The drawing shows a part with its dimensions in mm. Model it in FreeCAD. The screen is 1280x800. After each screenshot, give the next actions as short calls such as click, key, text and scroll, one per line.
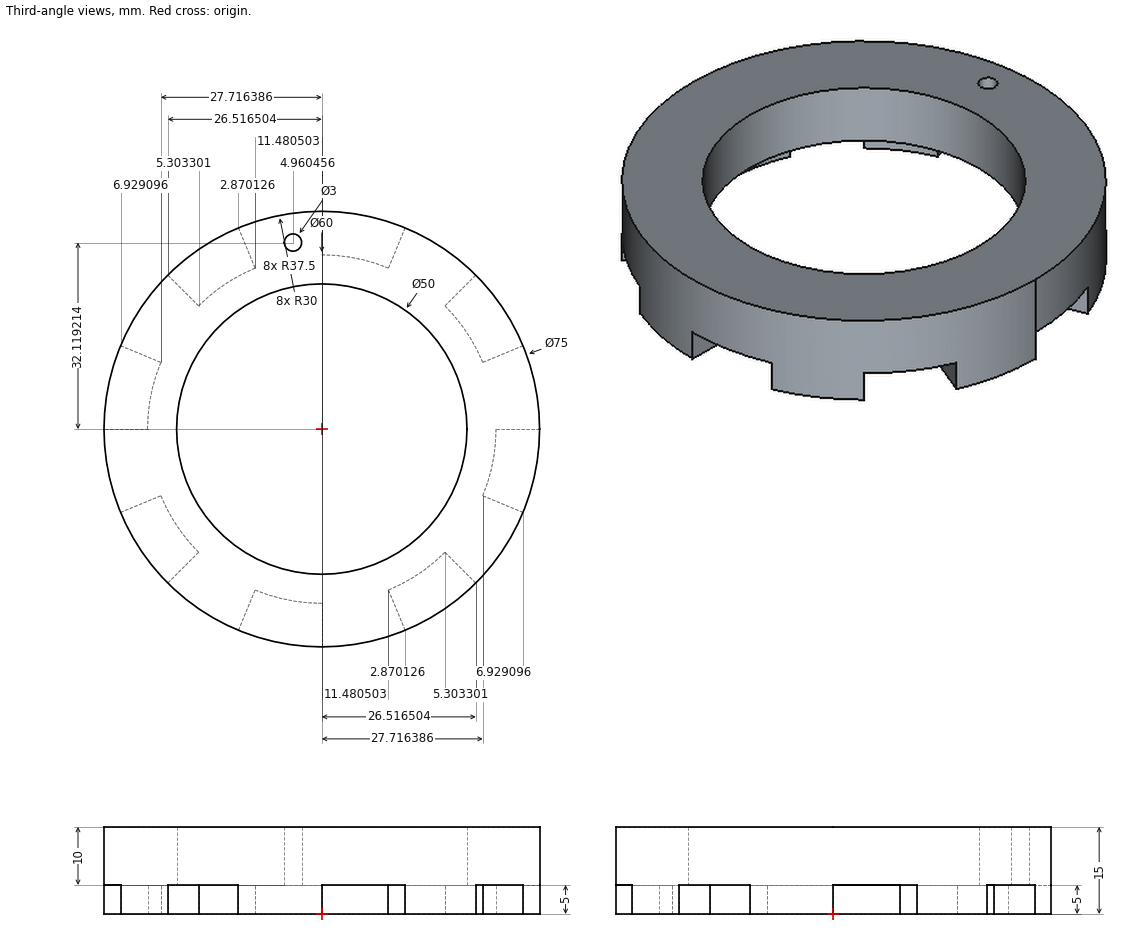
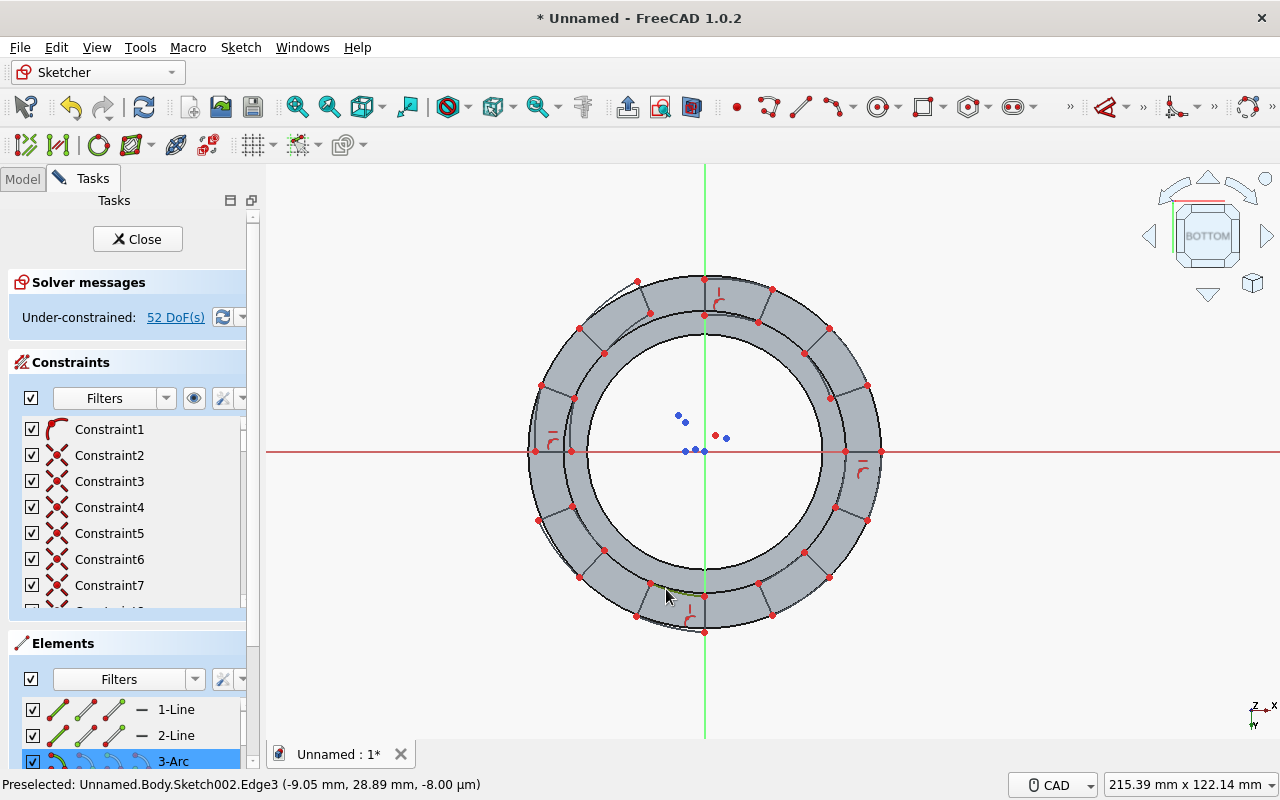
click(859, 367)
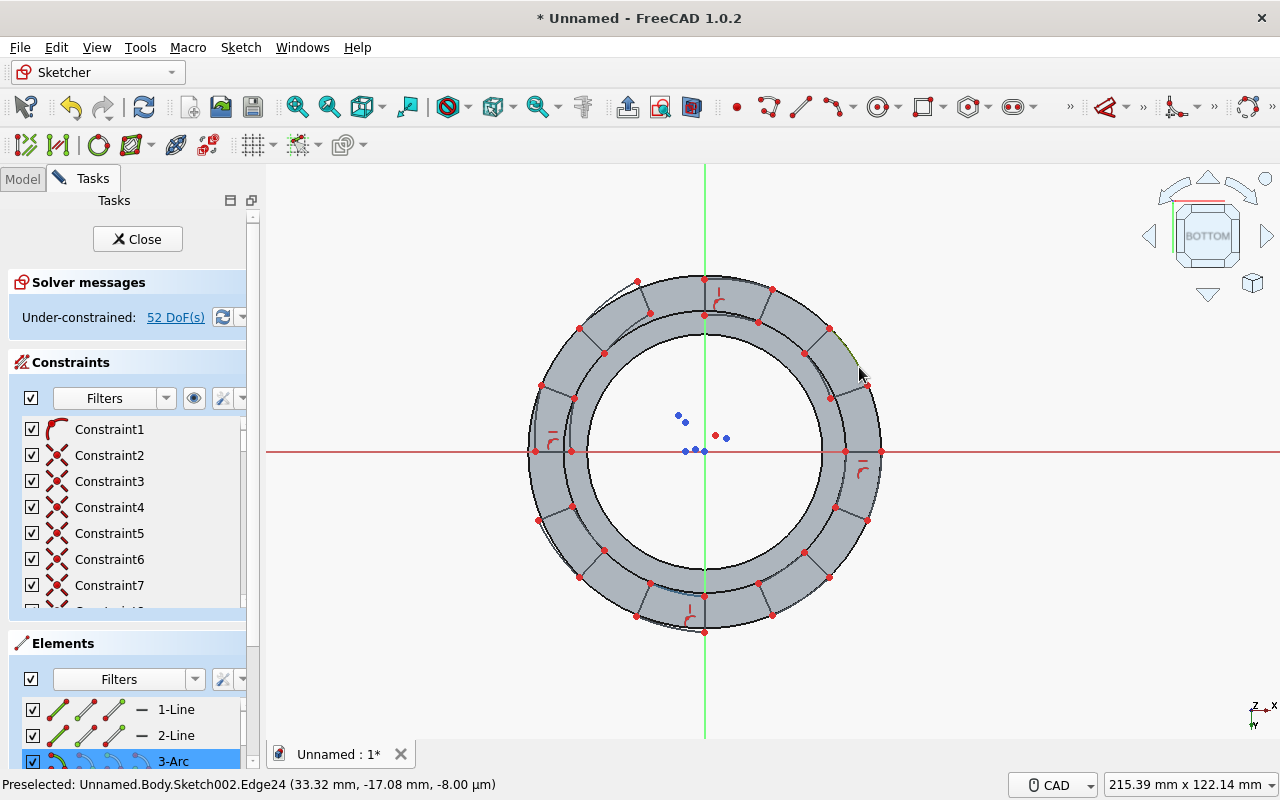
key(c)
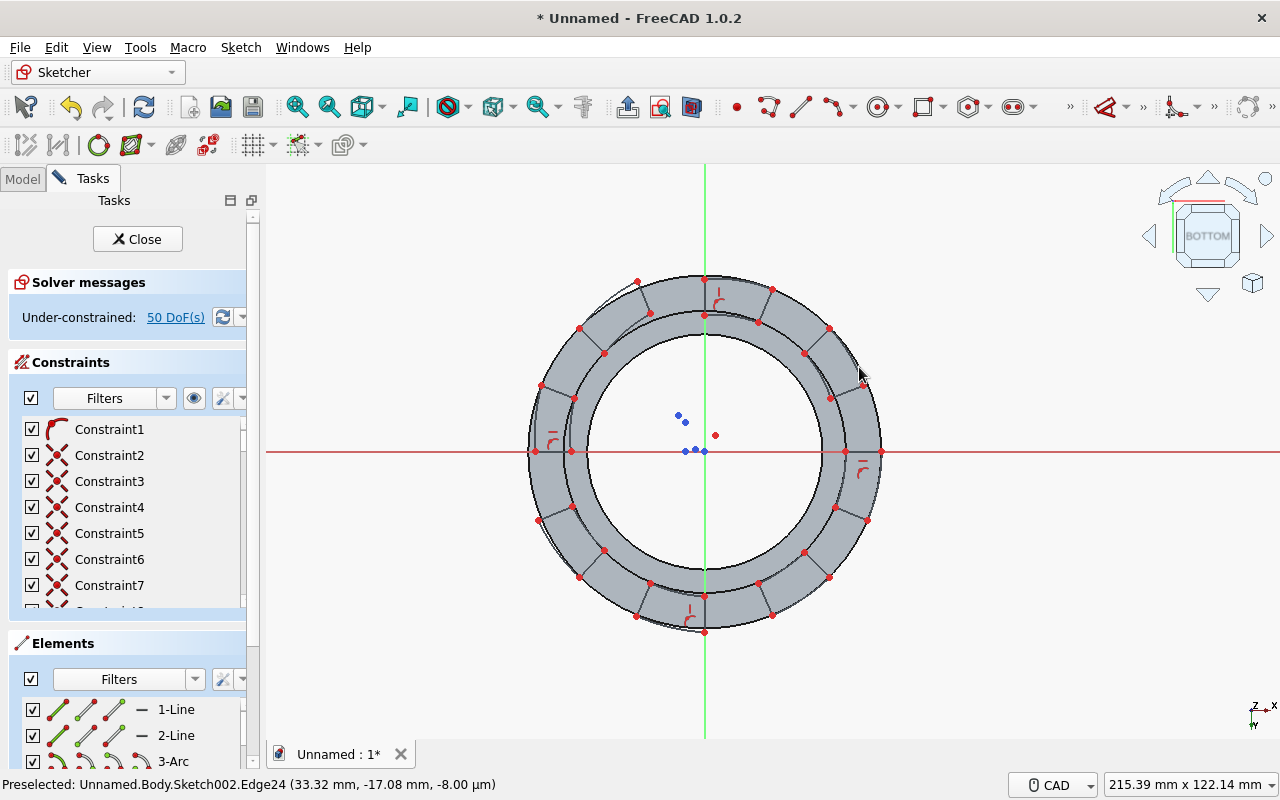
click(666, 589)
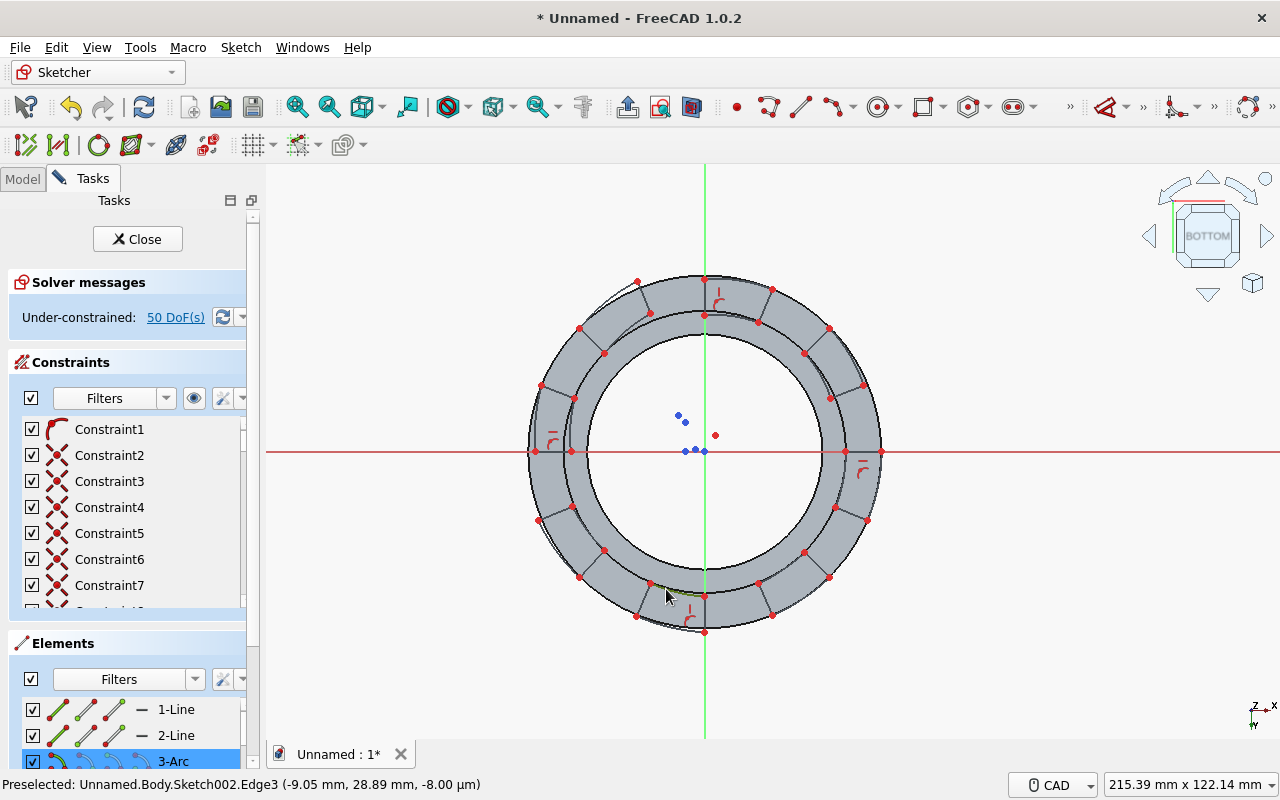
click(841, 491)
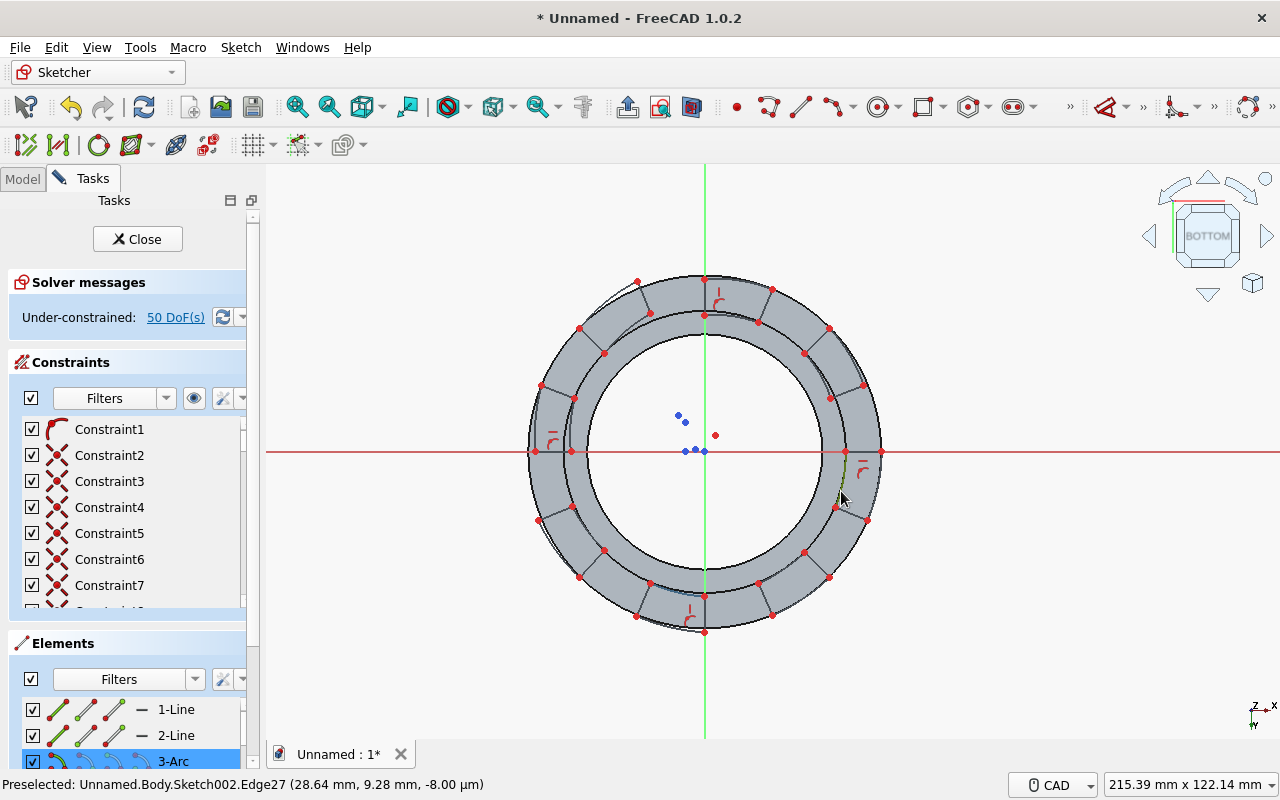
key(c)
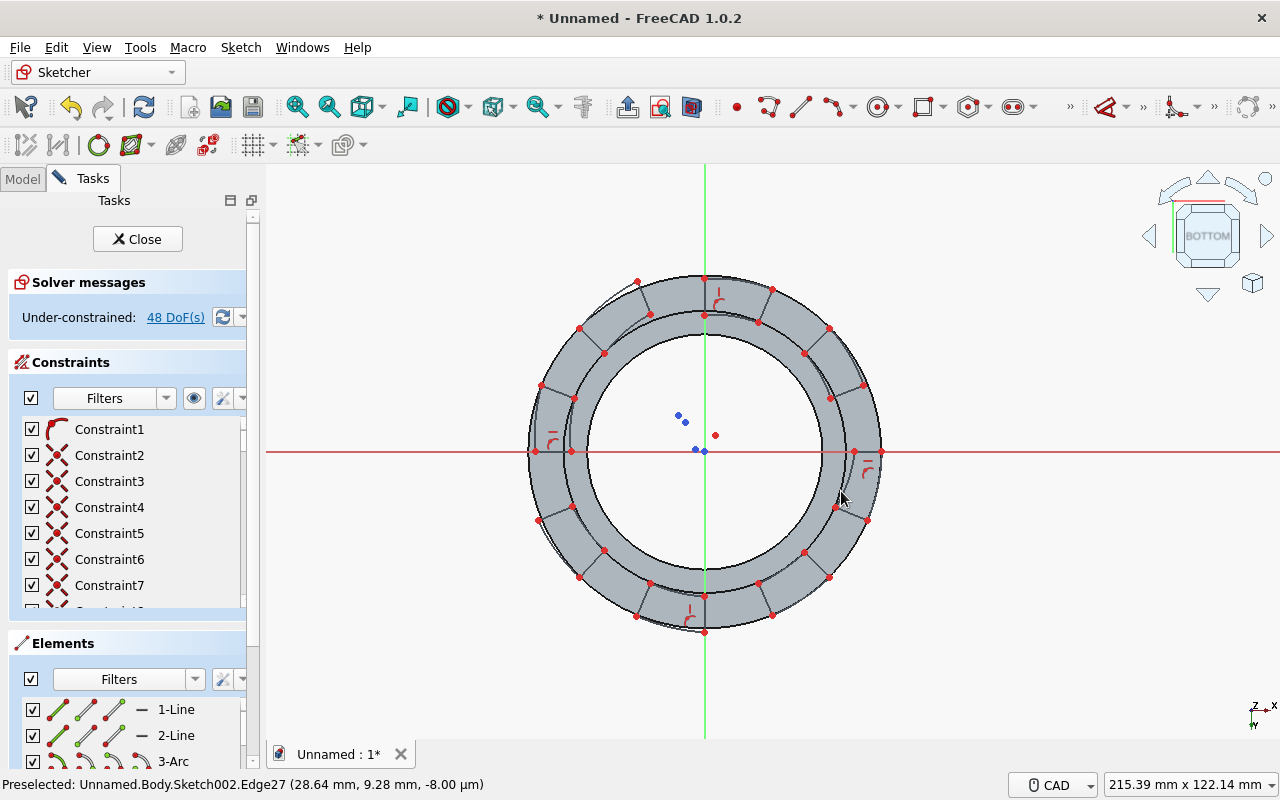
click(666, 589)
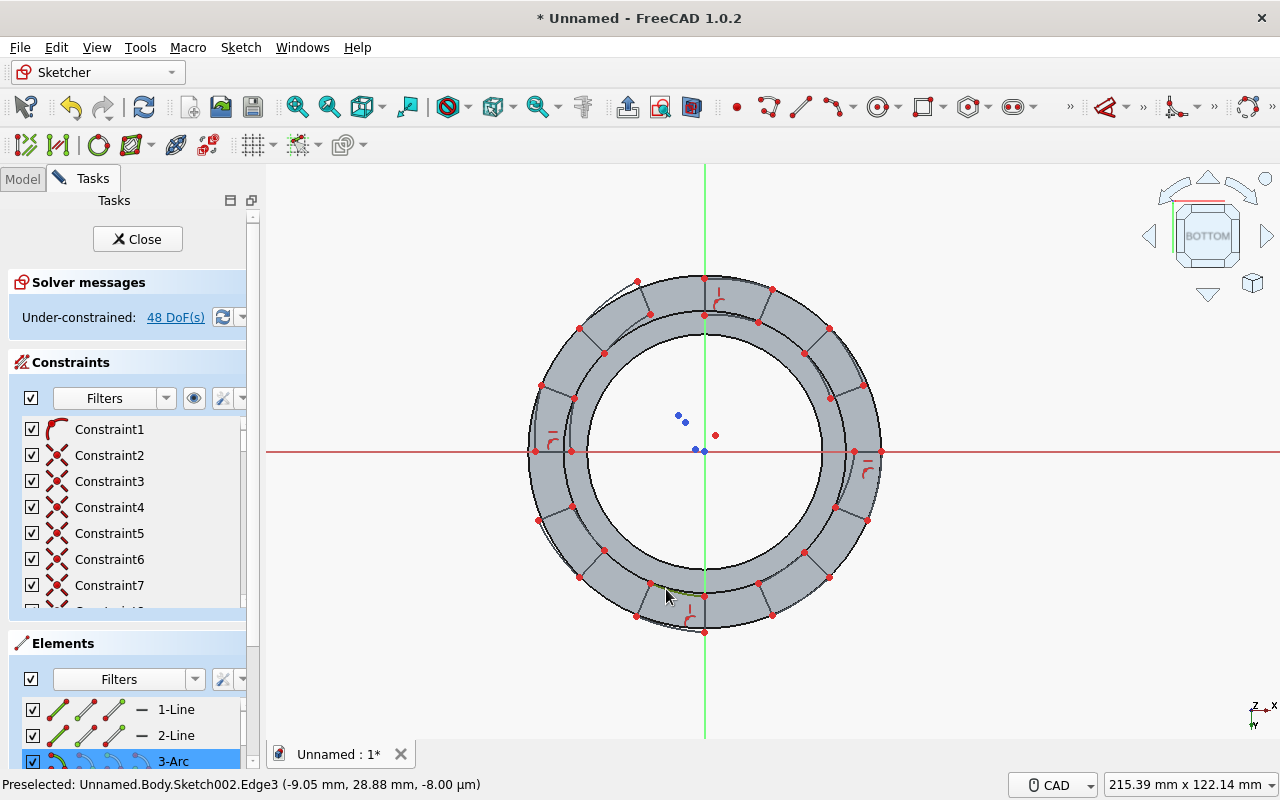
click(875, 501)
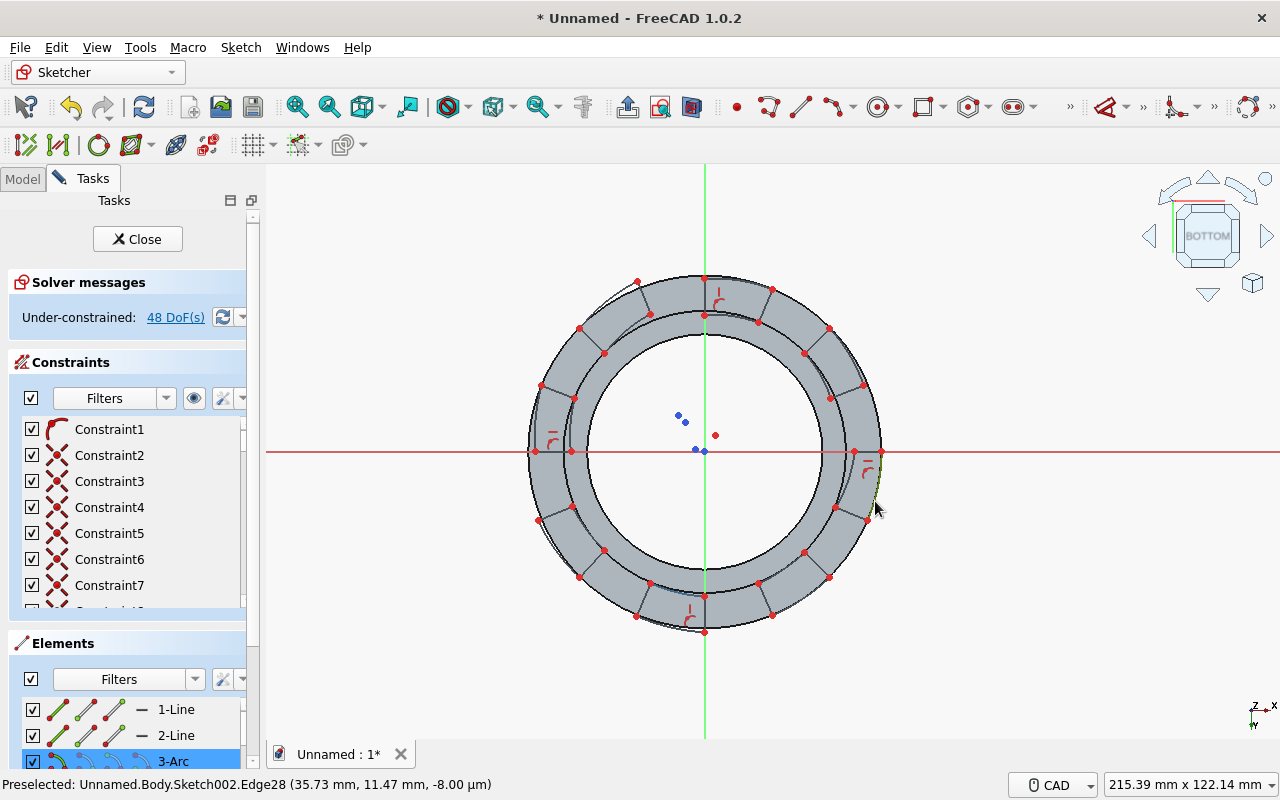
key(c)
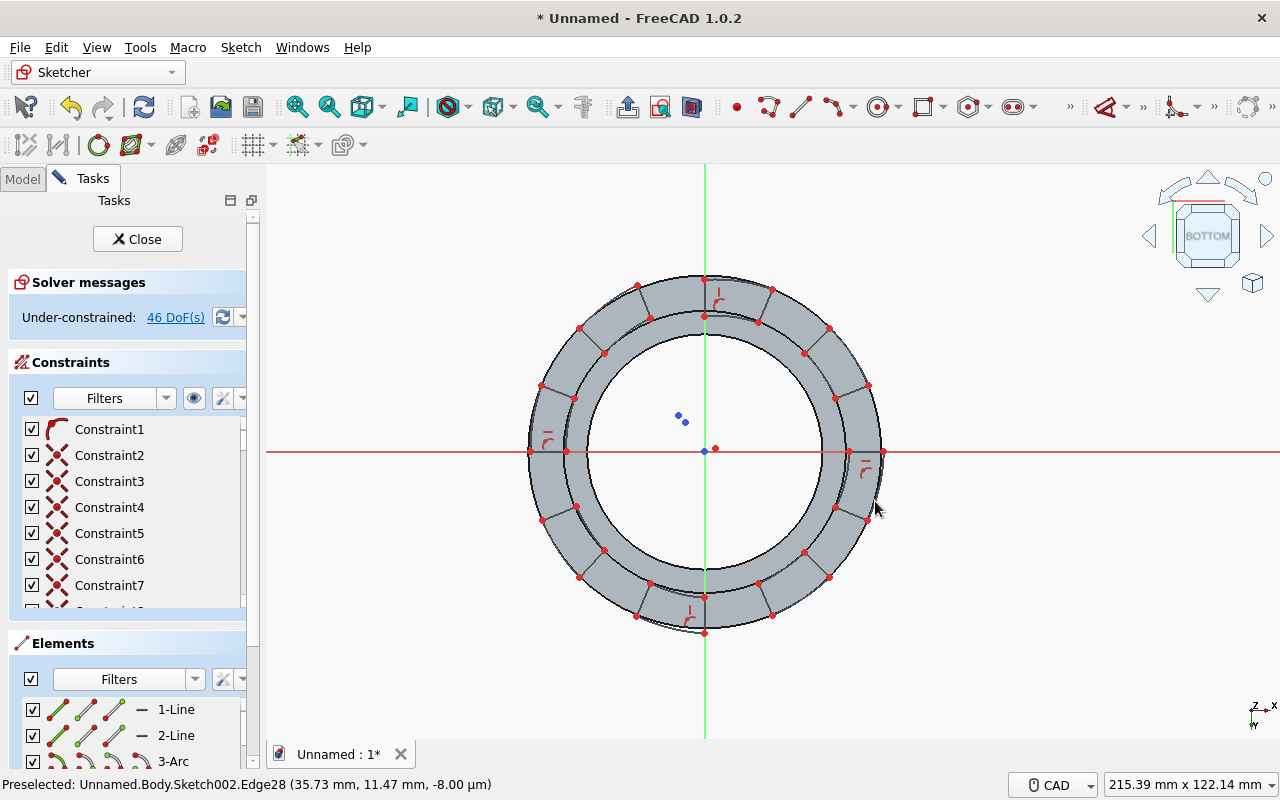
click(666, 590)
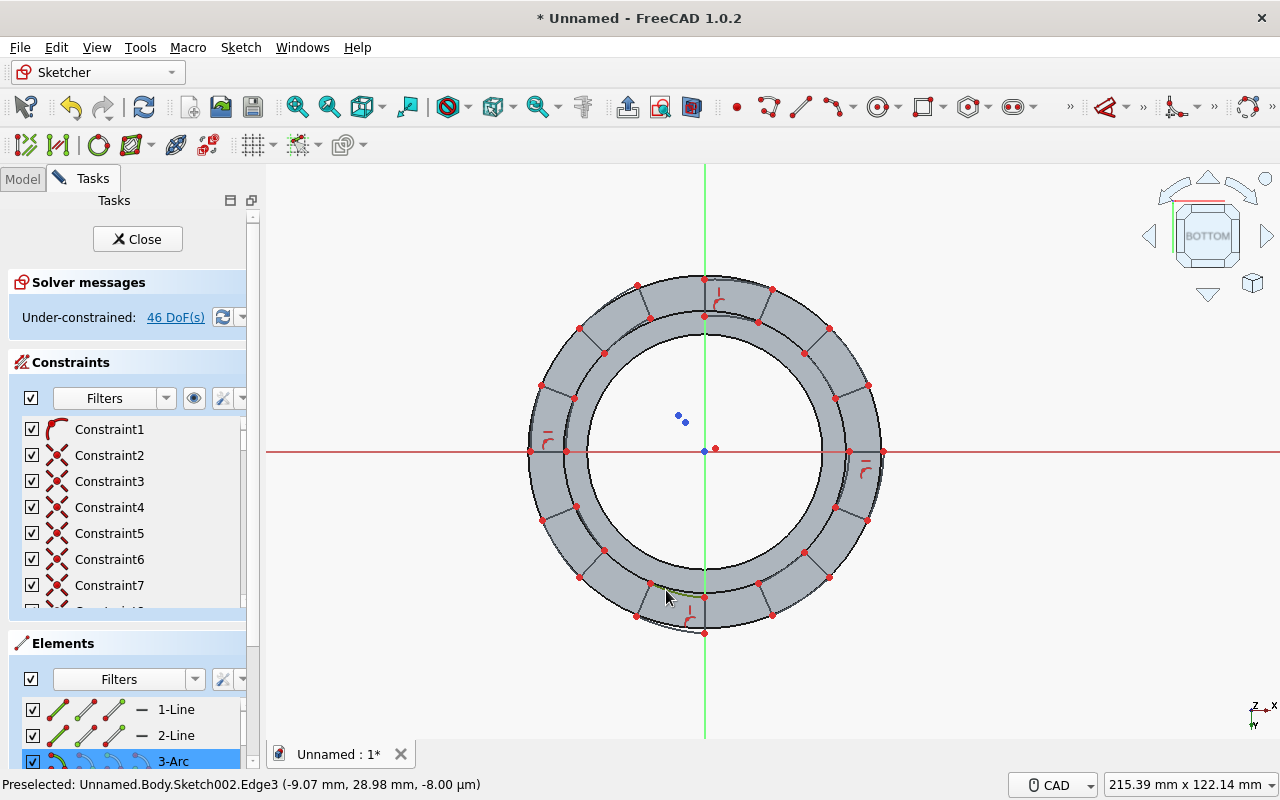
click(773, 576)